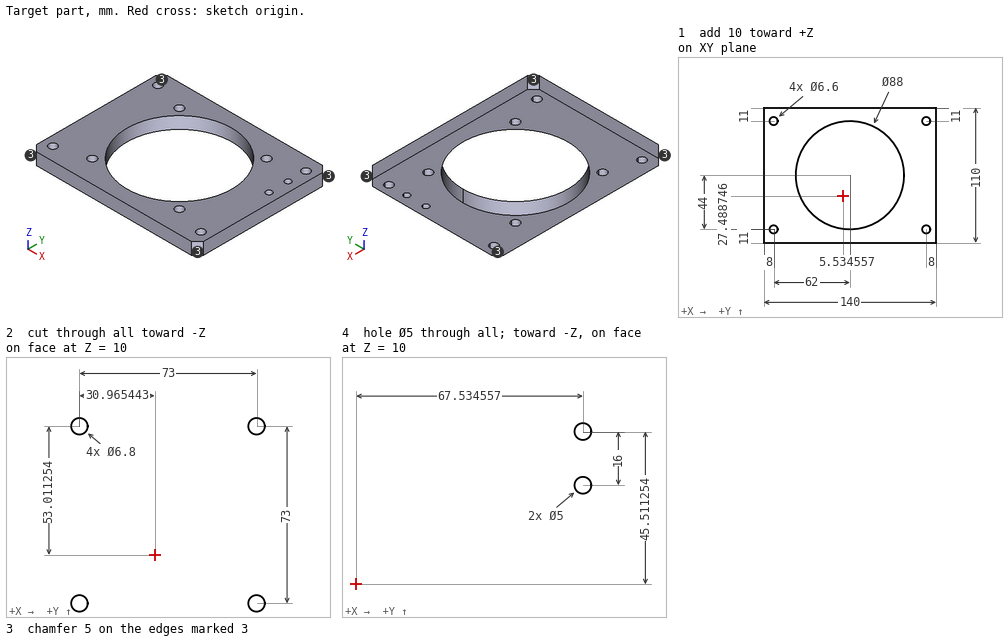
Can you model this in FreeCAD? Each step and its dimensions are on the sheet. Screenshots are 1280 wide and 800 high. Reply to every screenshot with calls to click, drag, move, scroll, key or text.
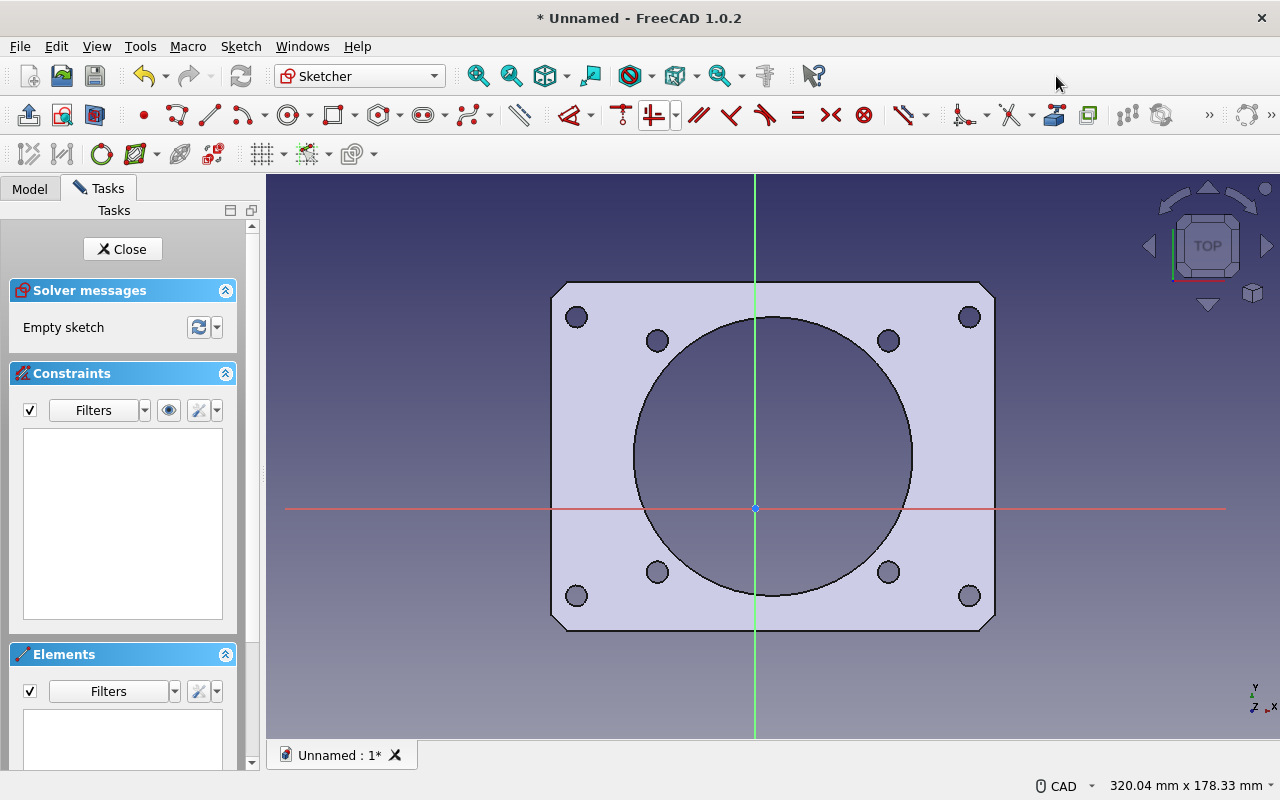
scroll(1036, 373, up, 8)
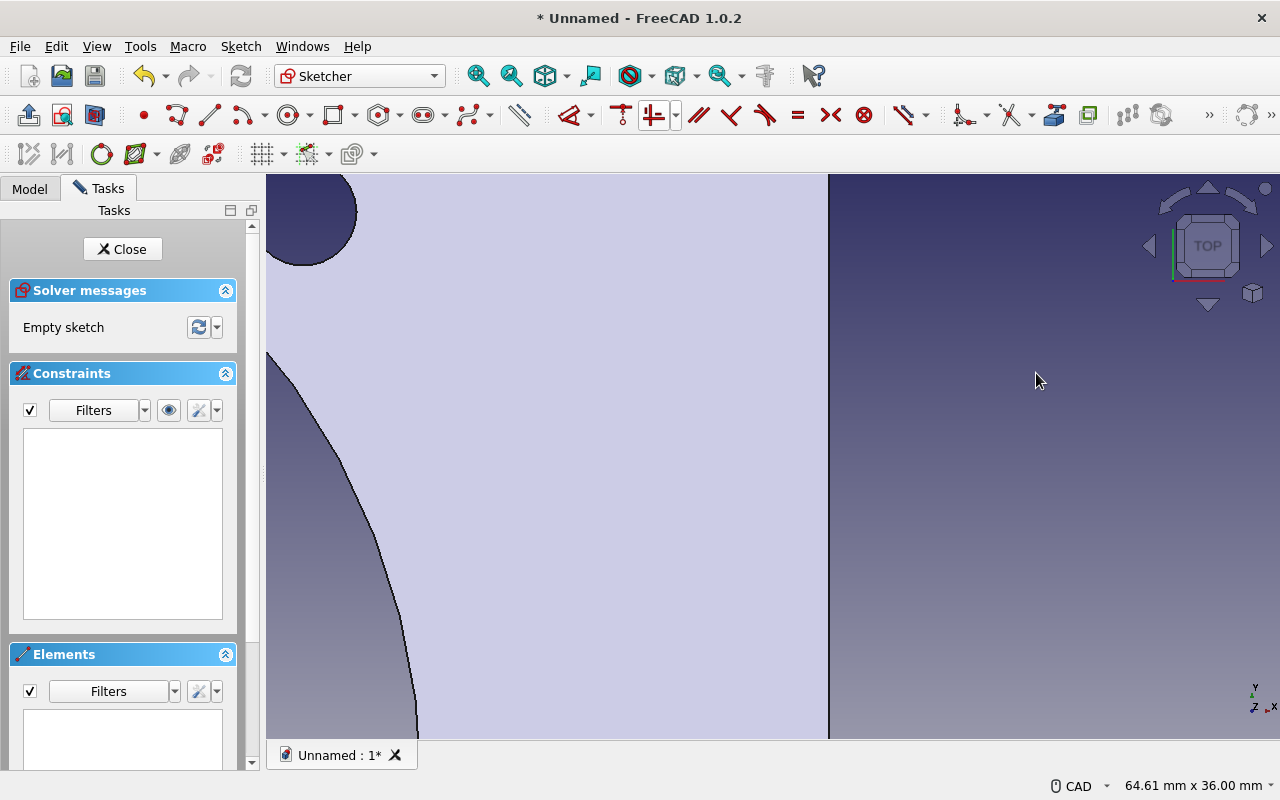
click(288, 116)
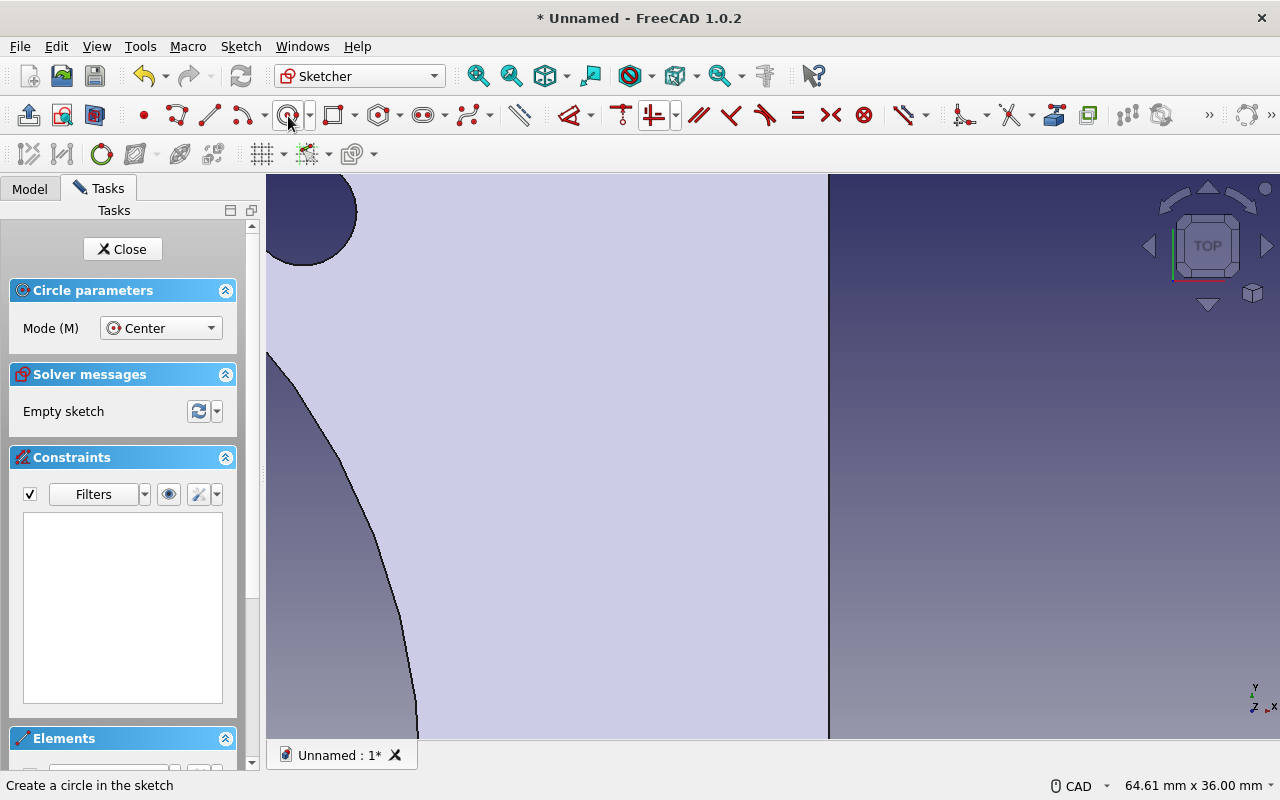
click(703, 330)
move(731, 302)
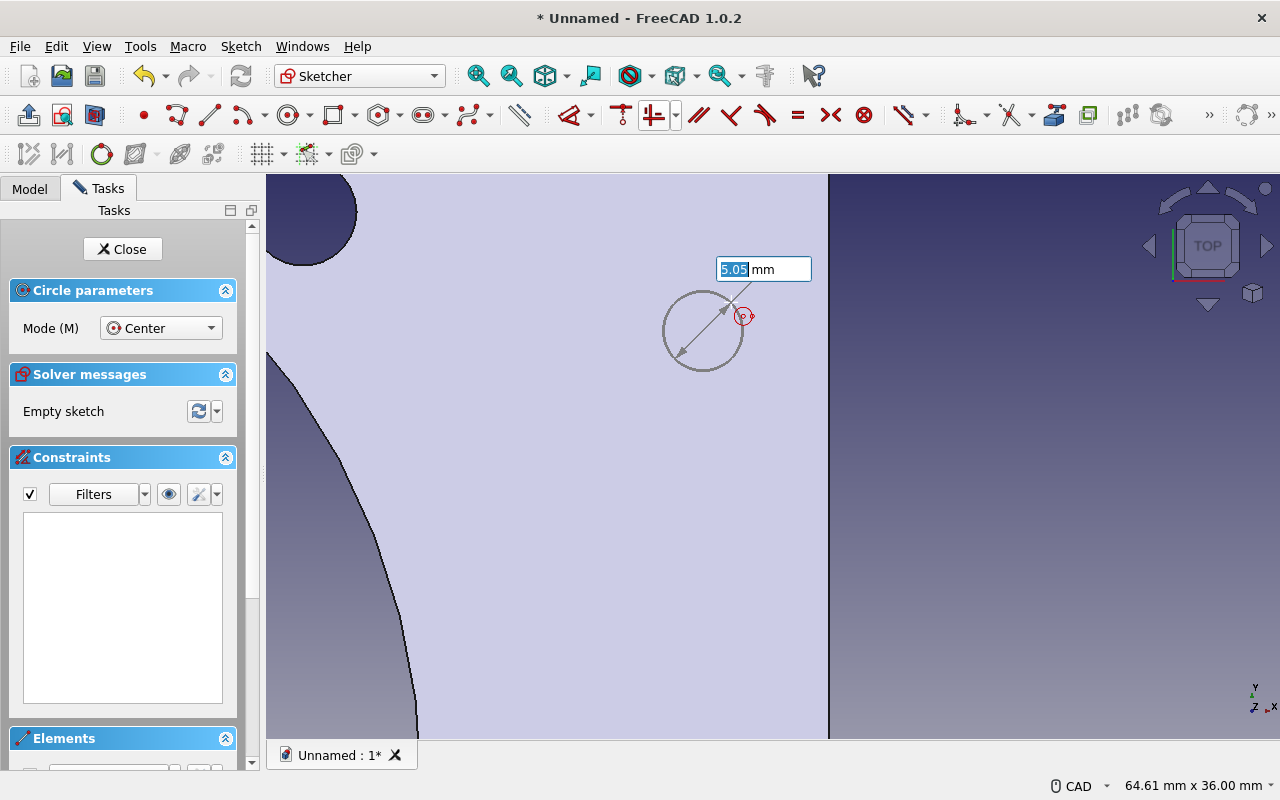
text(5)
key(Return)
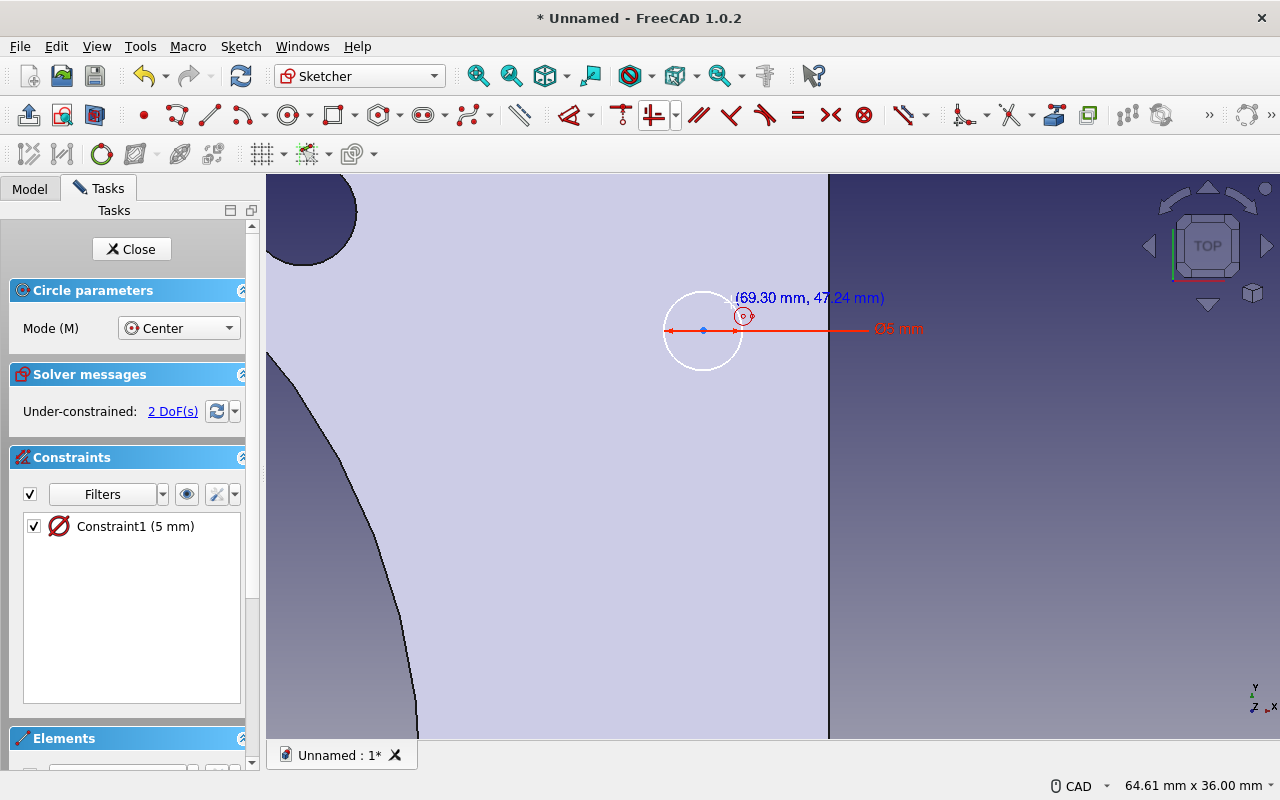
click(703, 581)
move(731, 553)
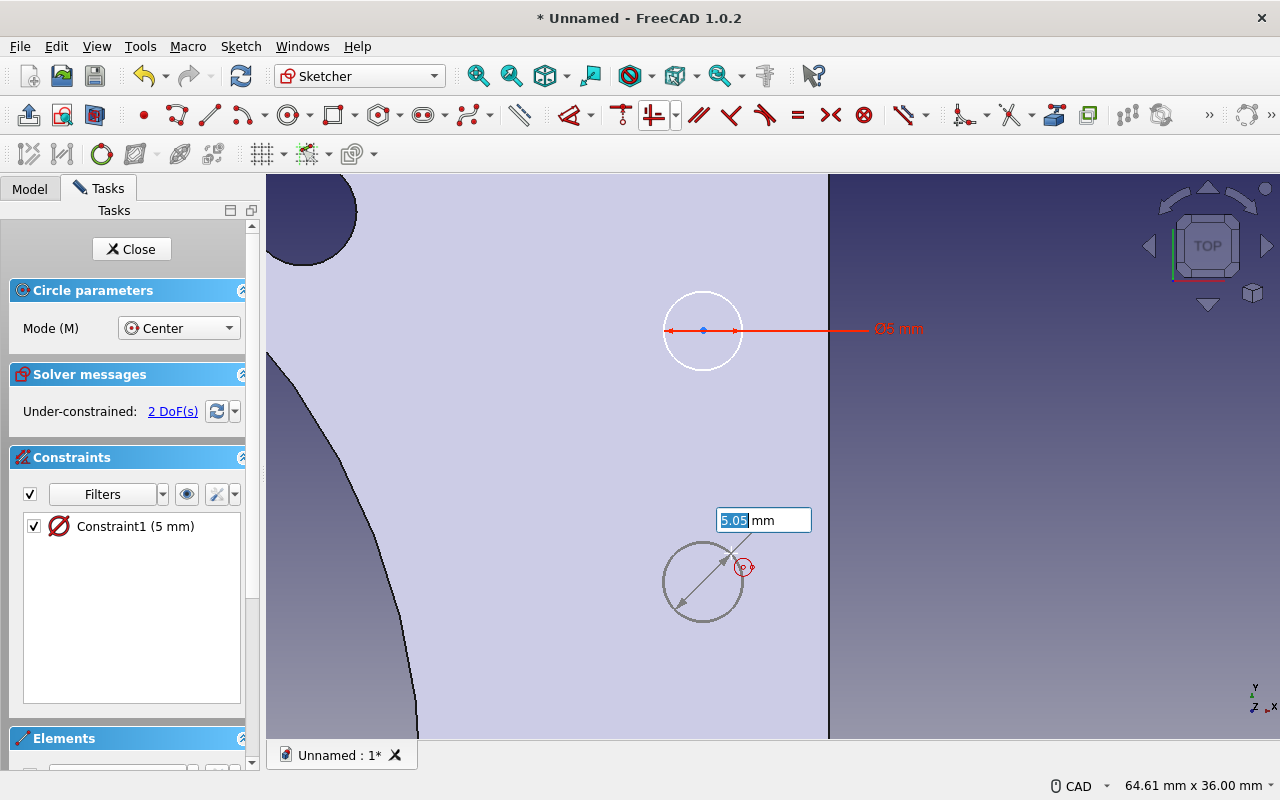
text(5)
key(Return)
key(Escape)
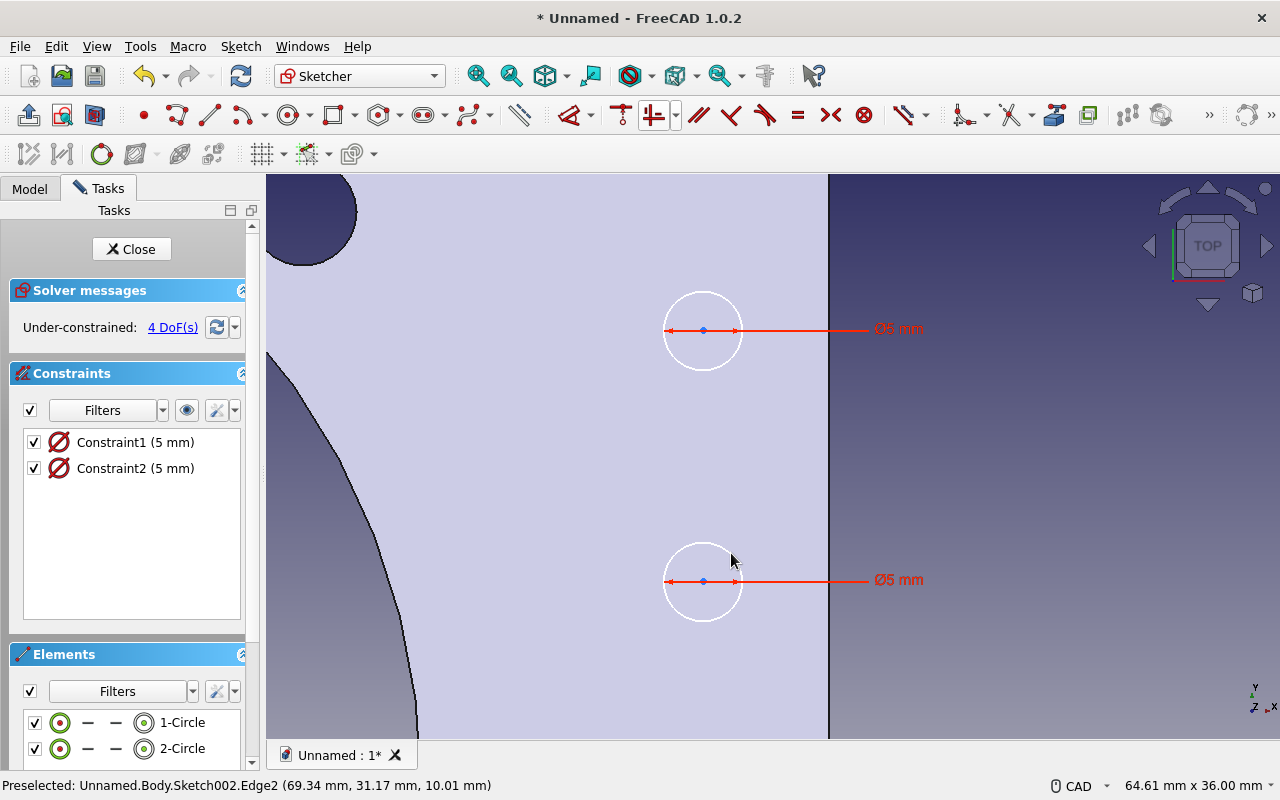
click(703, 331)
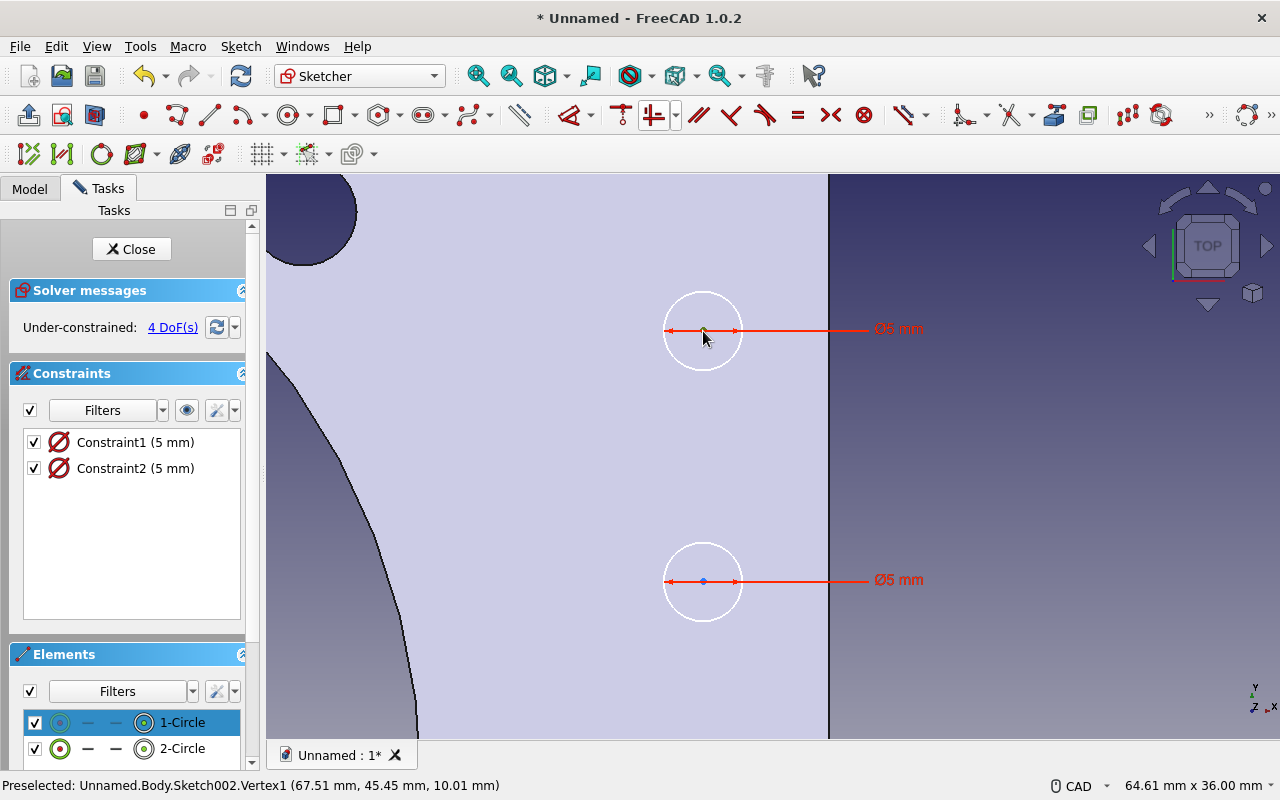
click(703, 582)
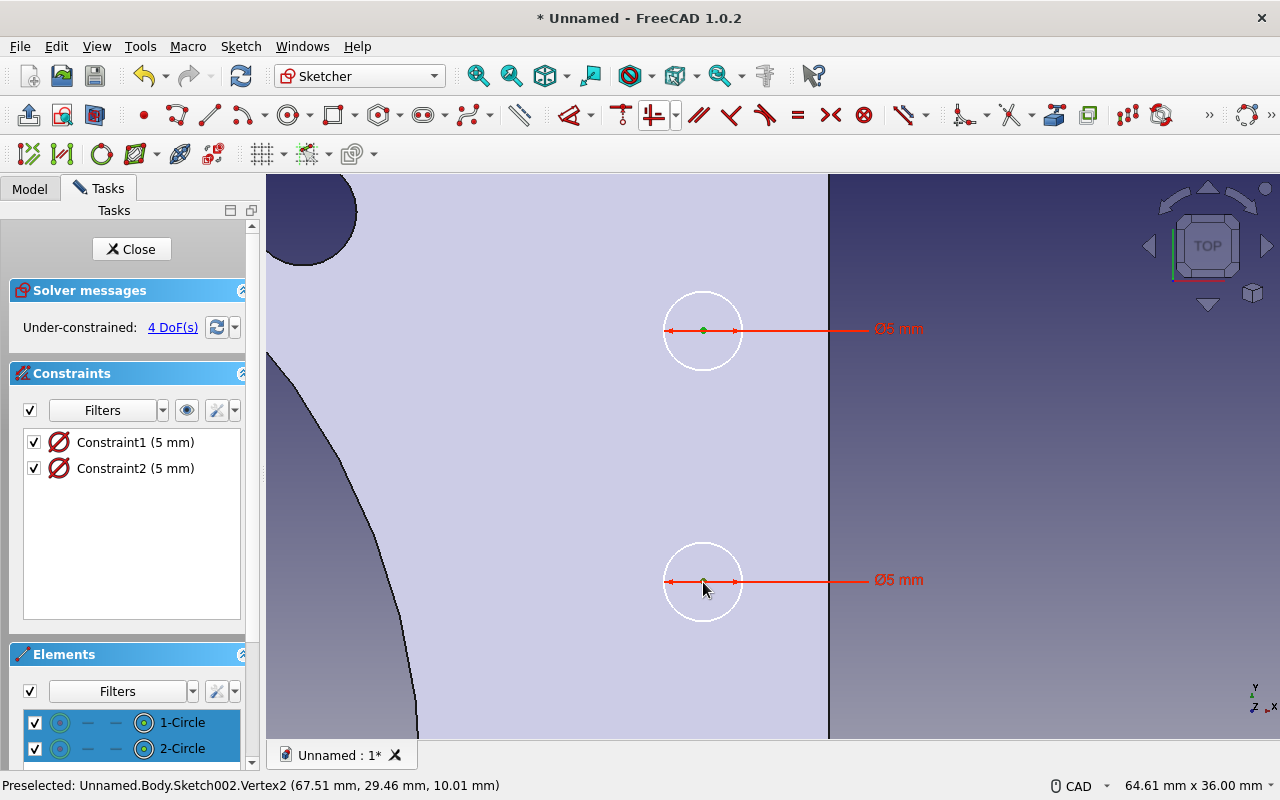
click(676, 116)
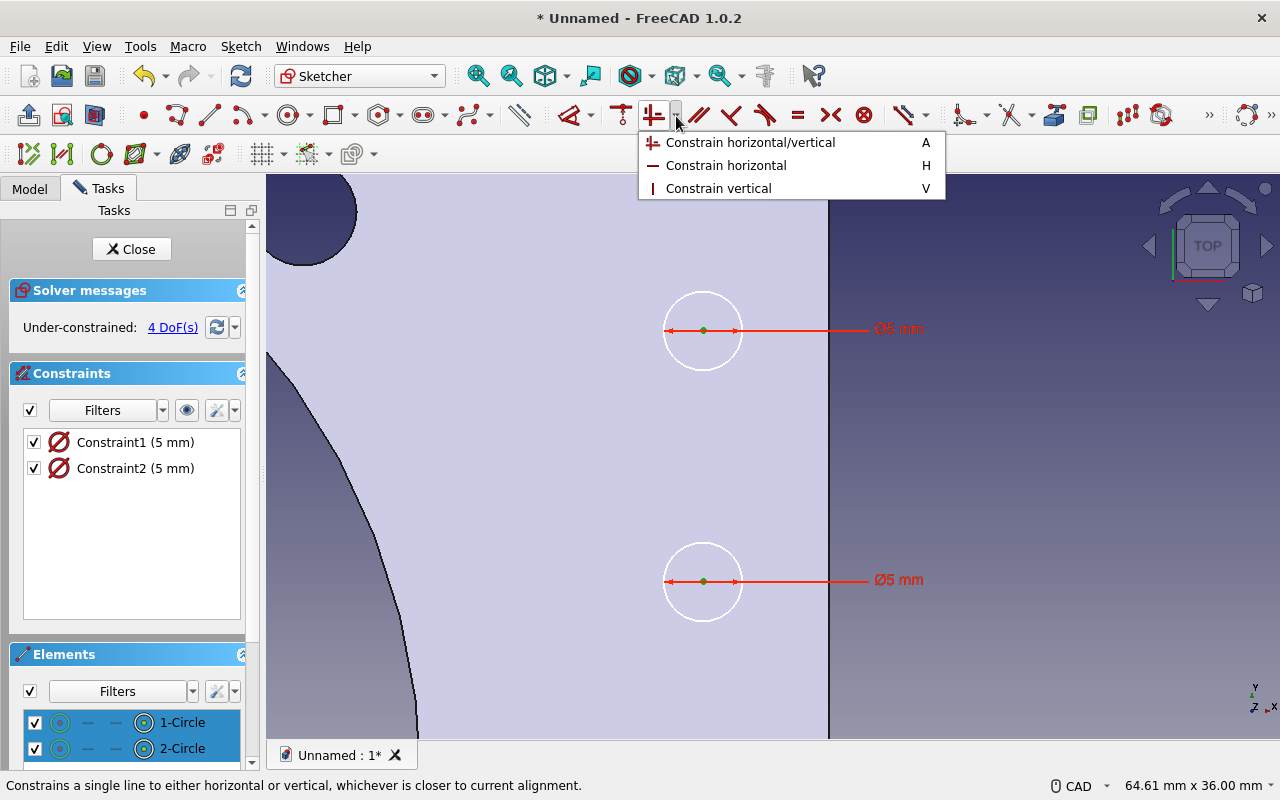
click(792, 188)